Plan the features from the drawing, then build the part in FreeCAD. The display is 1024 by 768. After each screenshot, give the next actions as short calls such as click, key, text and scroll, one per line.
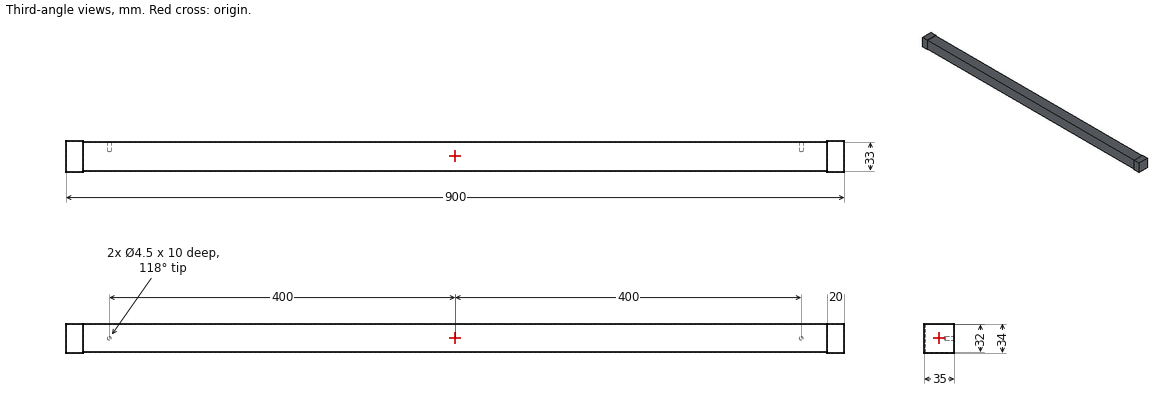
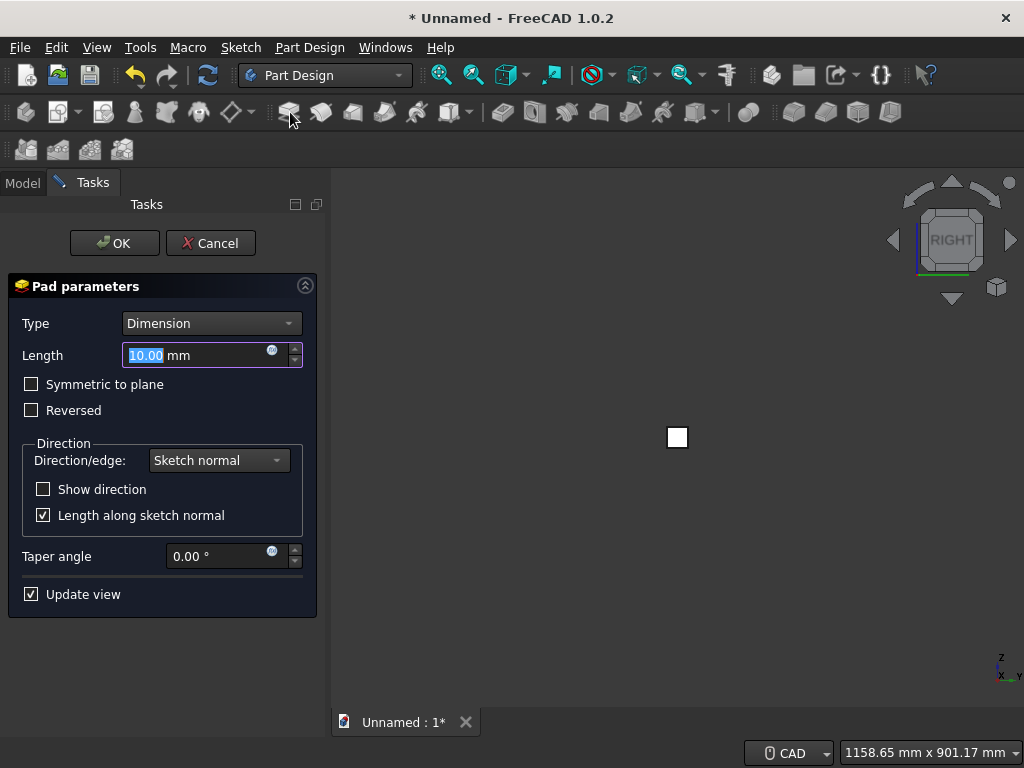
text(20)
key(Tab)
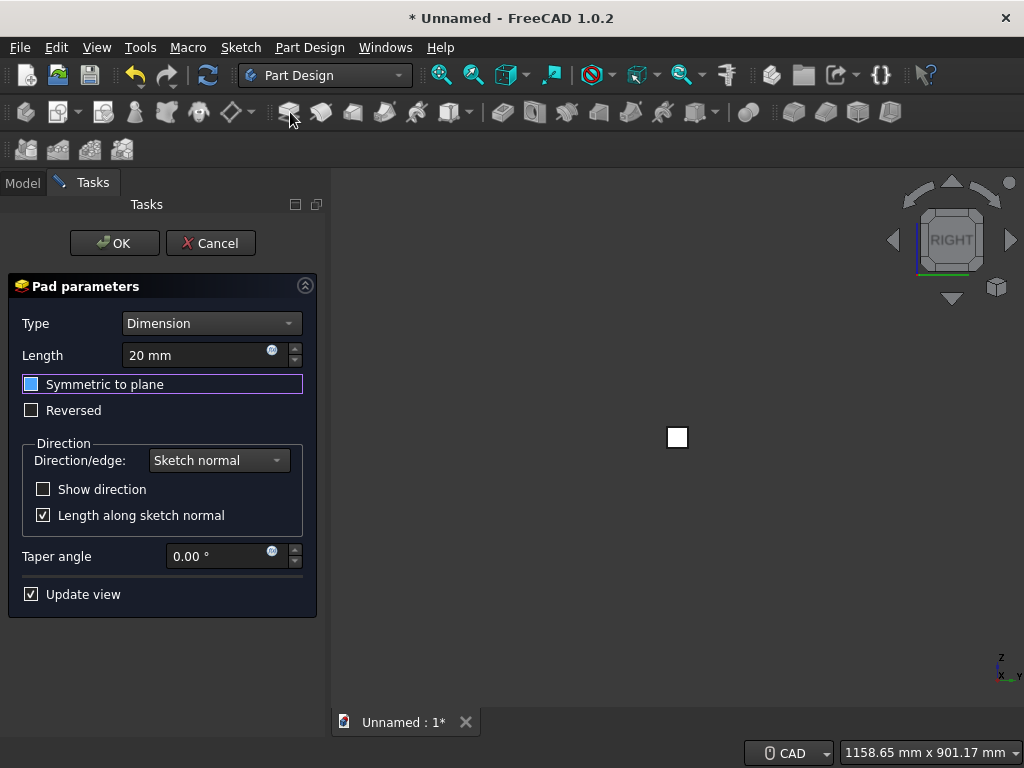
click(30, 410)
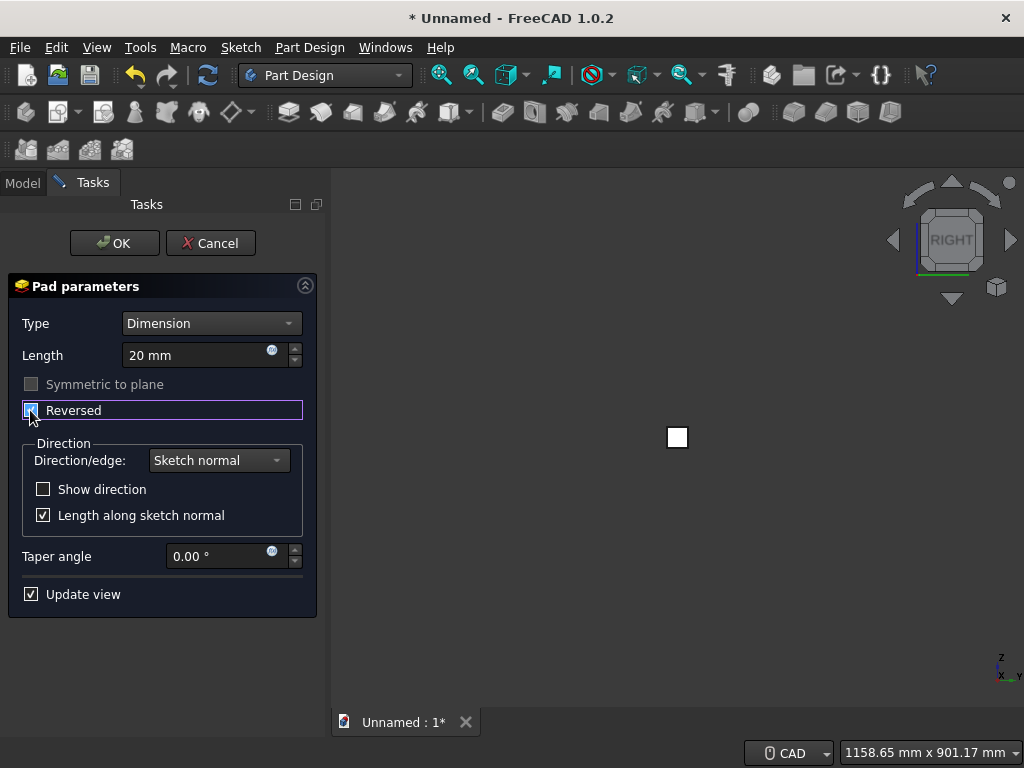
click(115, 243)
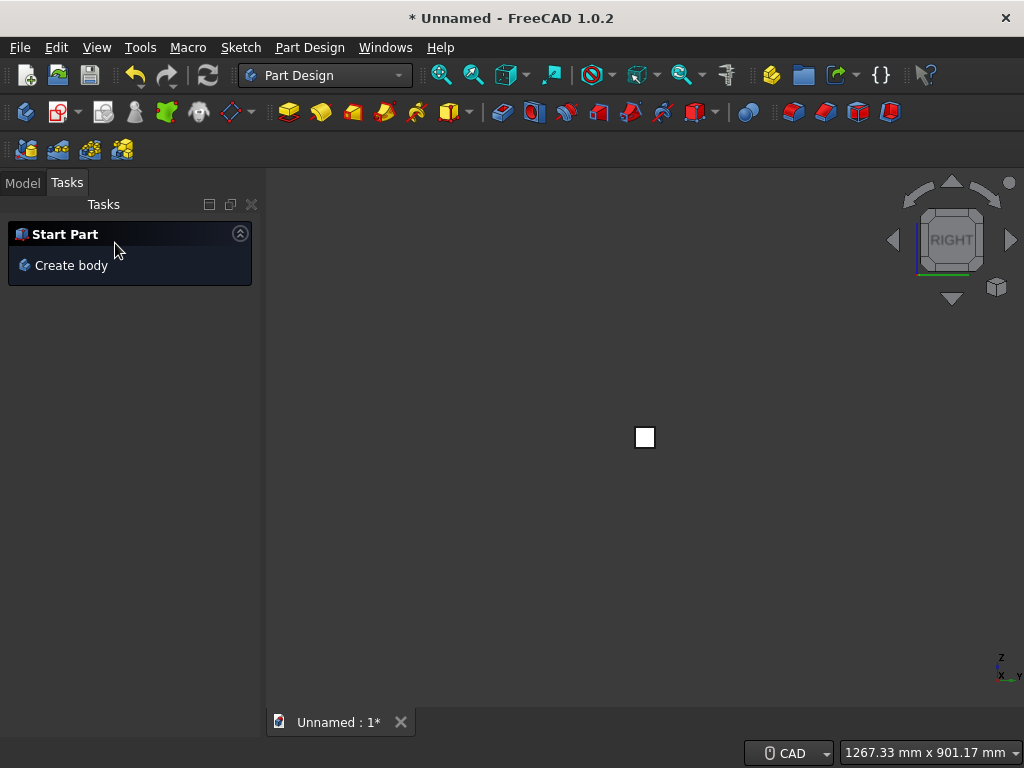
click(442, 76)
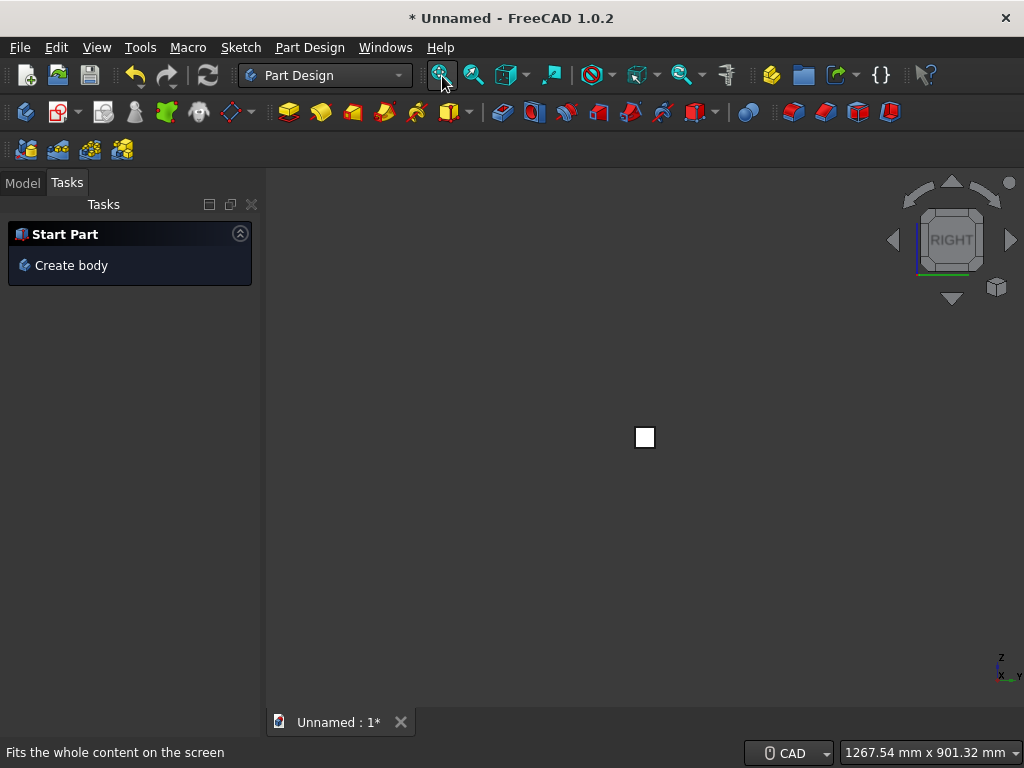
click(23, 182)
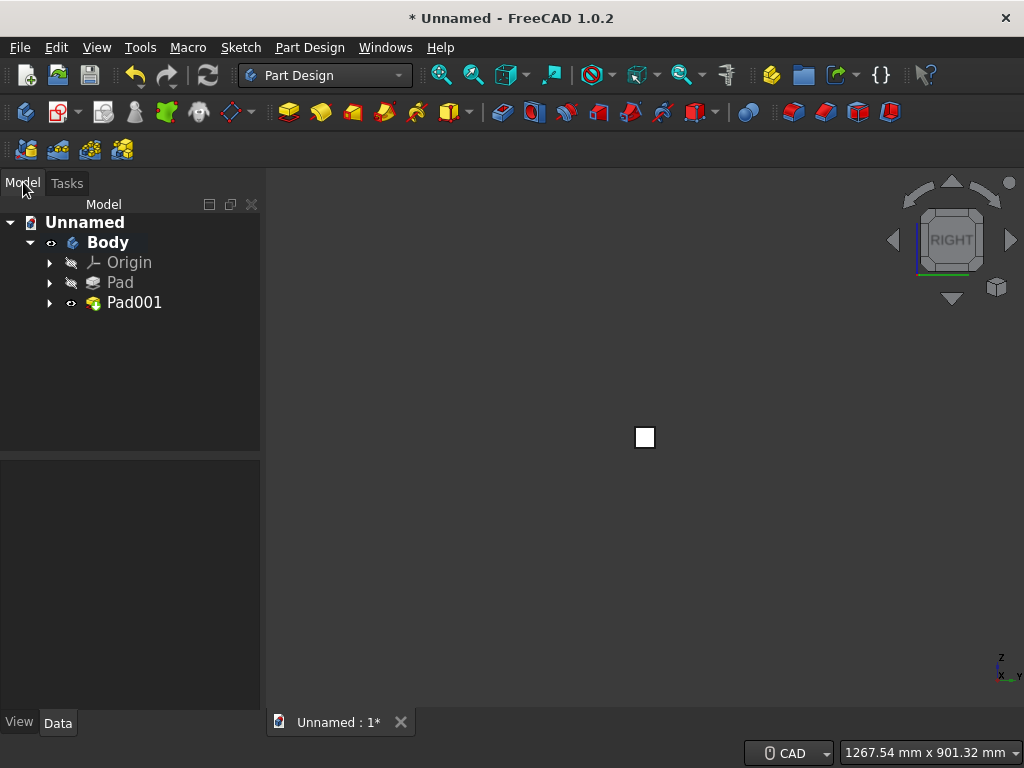
click(116, 303)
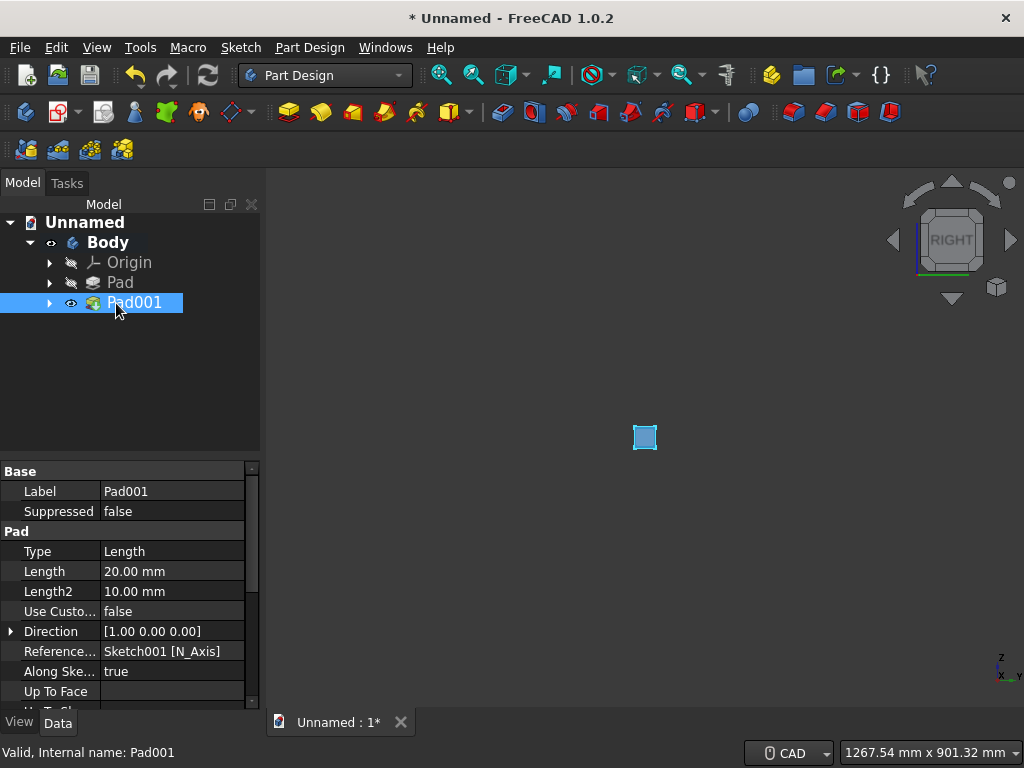
click(26, 150)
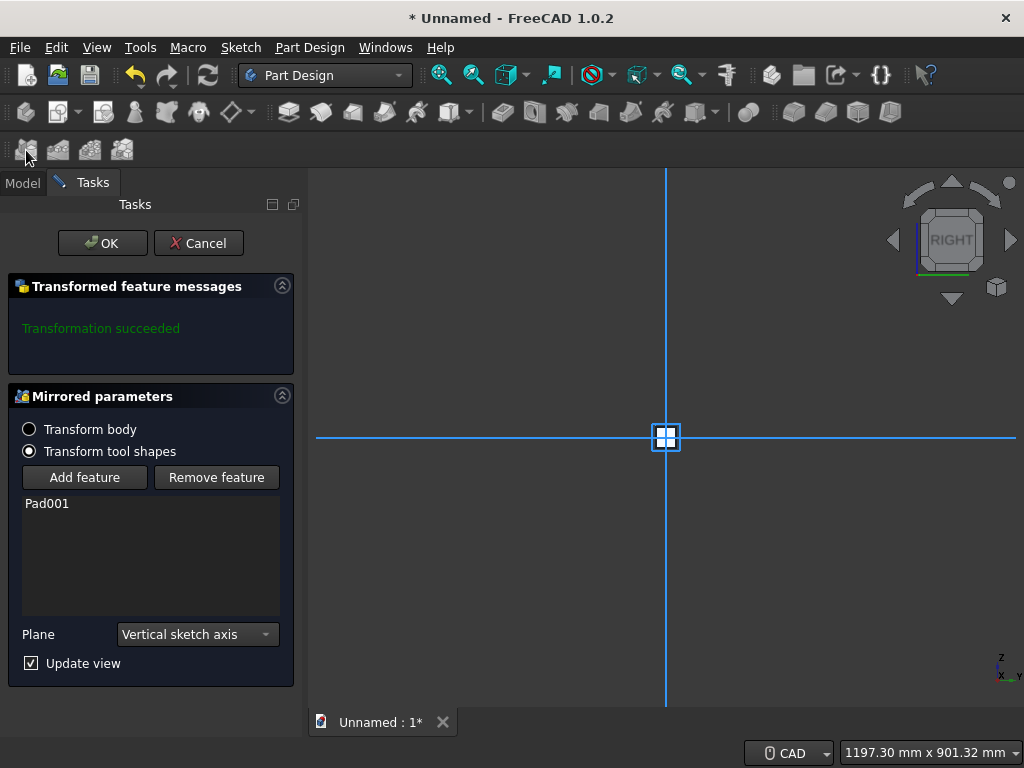
click(198, 634)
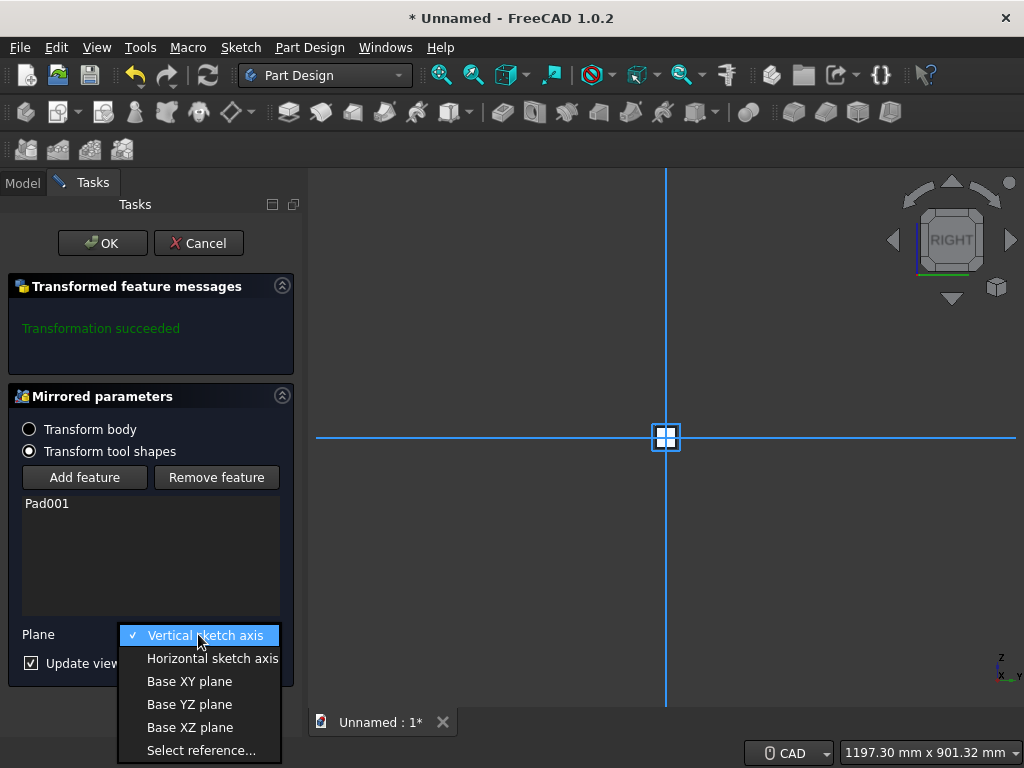
click(198, 704)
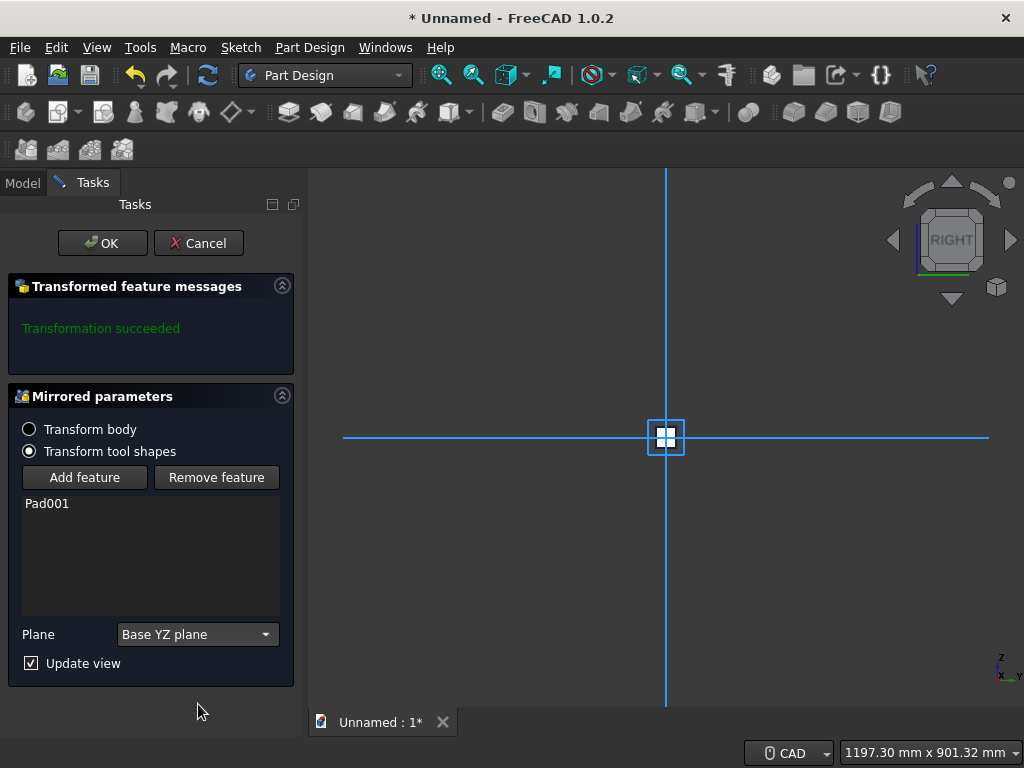
click(103, 243)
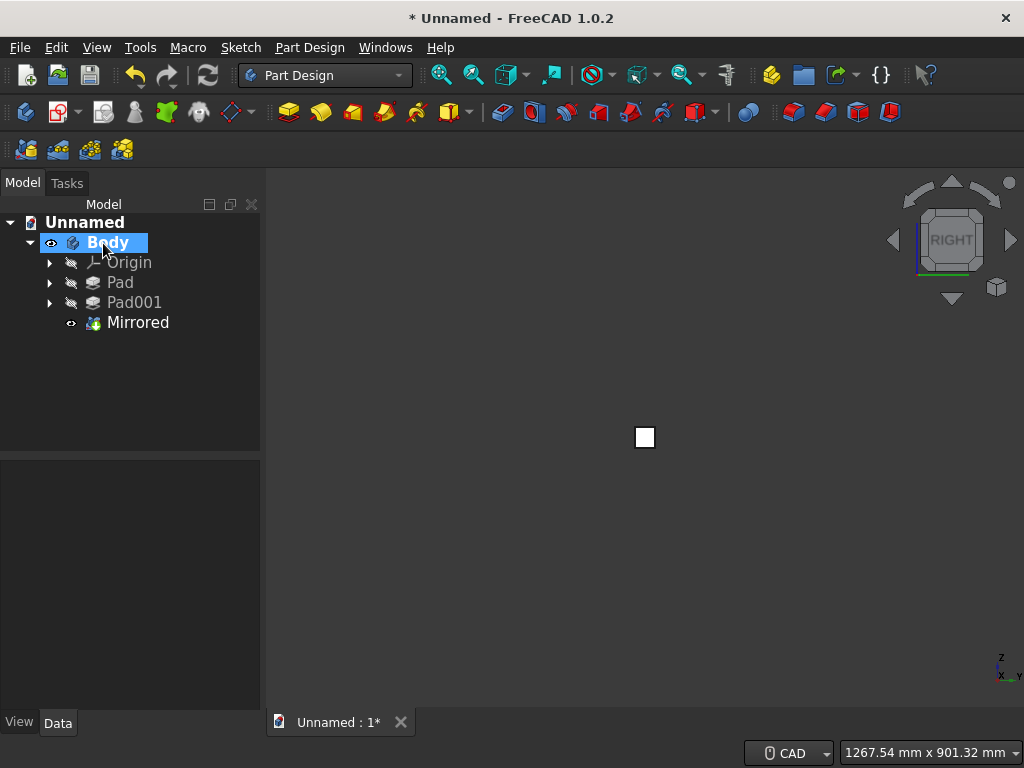
key(v)
key(f)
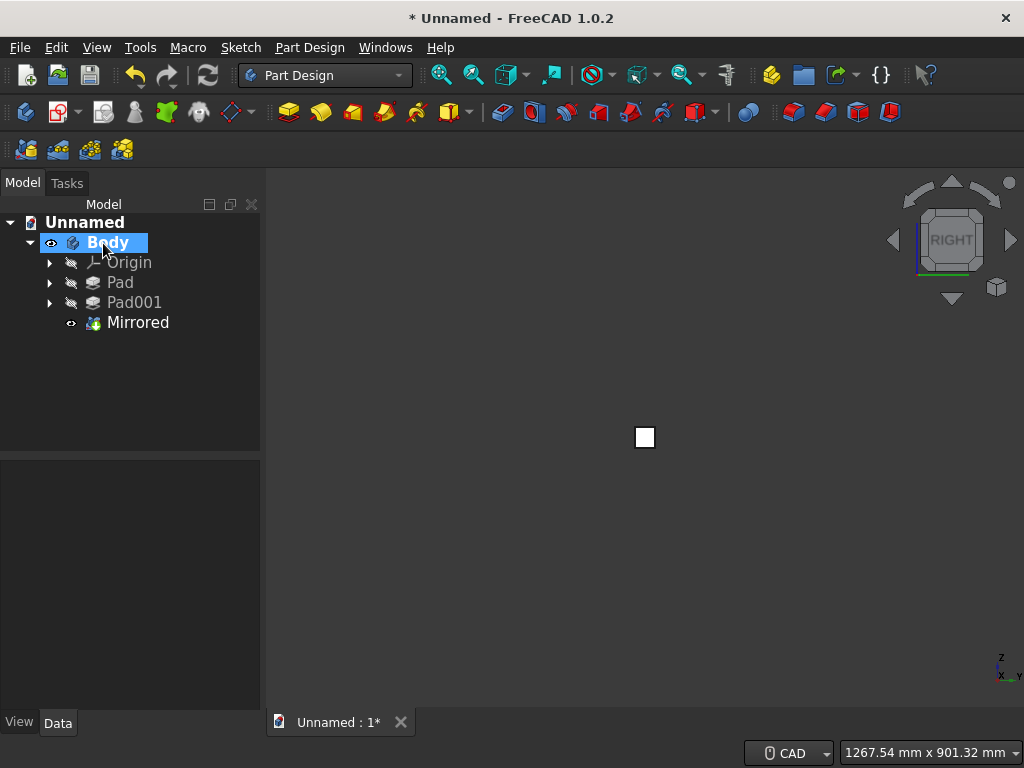
key(4)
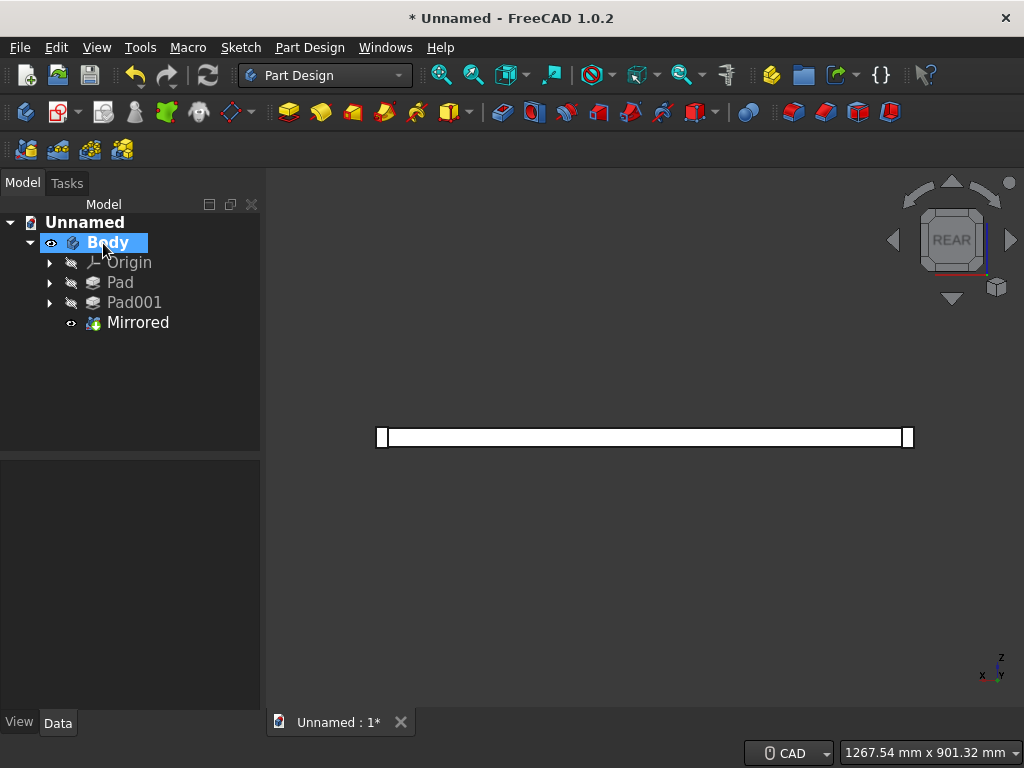
click(425, 436)